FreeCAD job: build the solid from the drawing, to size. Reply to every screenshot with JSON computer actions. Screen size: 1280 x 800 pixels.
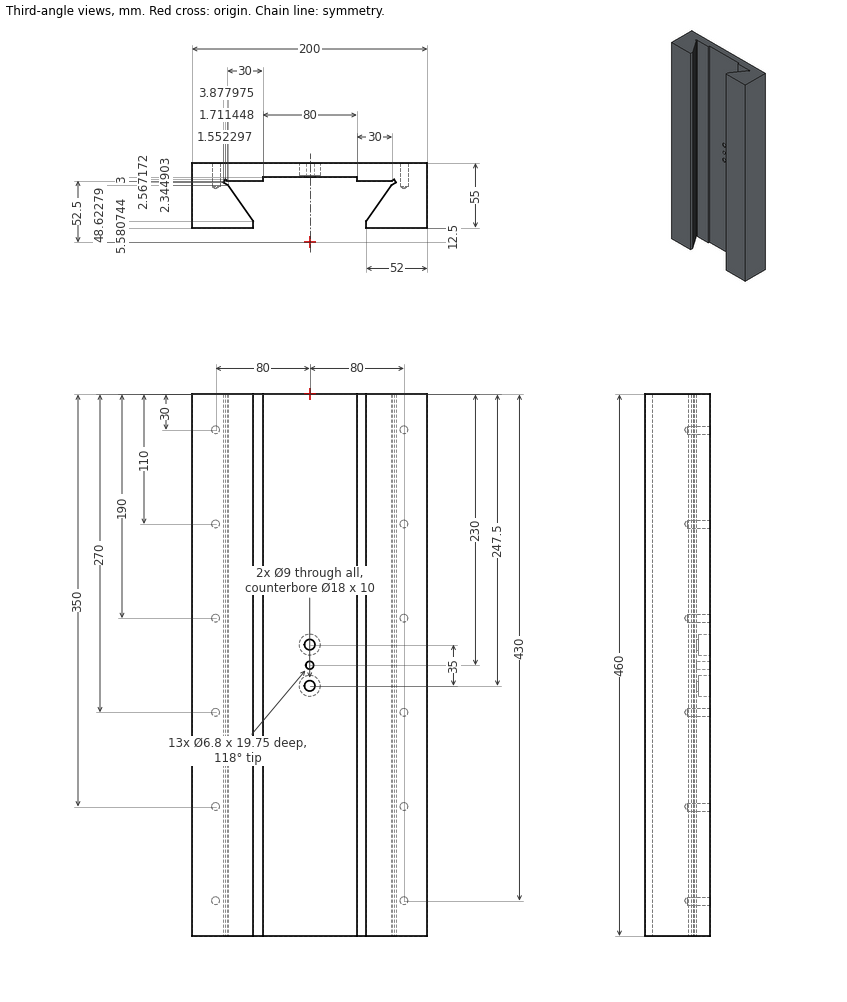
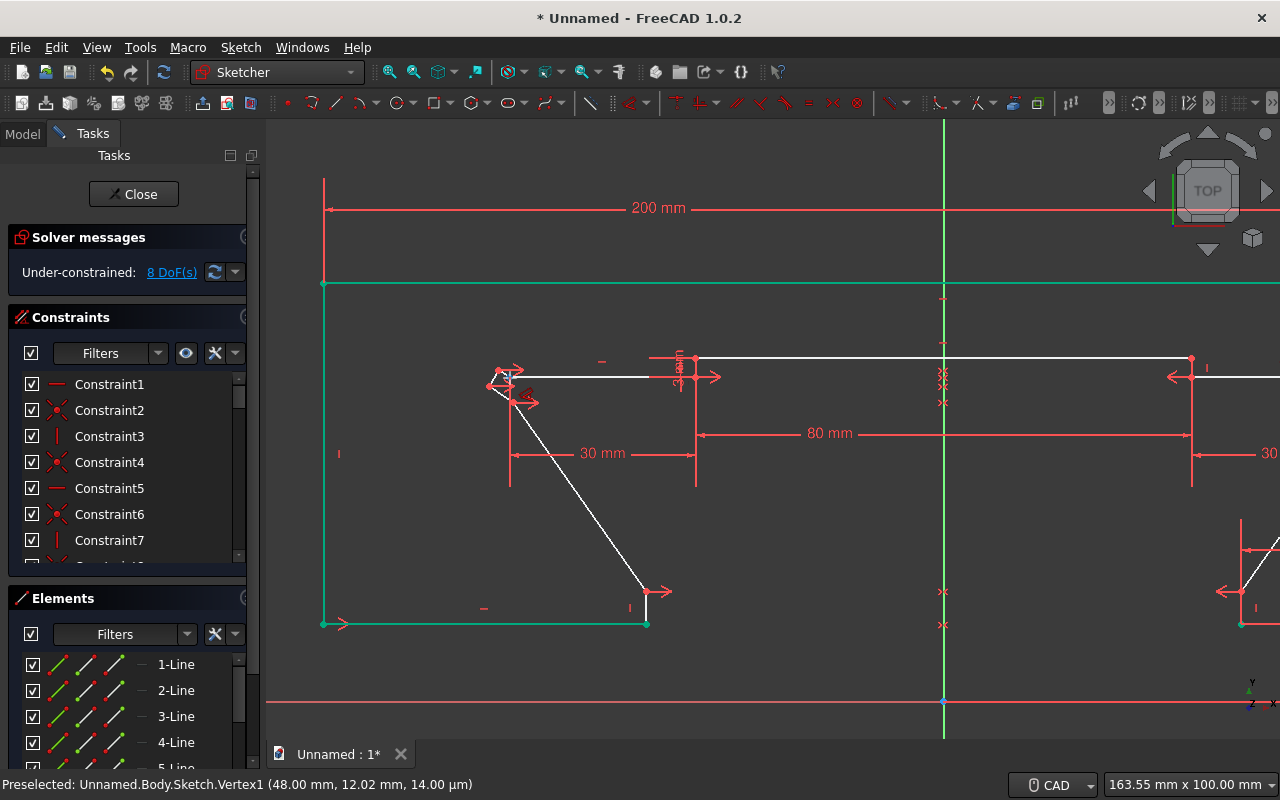
{"action": "left_click", "coordinate": [510, 377]}
{"action": "left_click", "coordinate": [476, 539]}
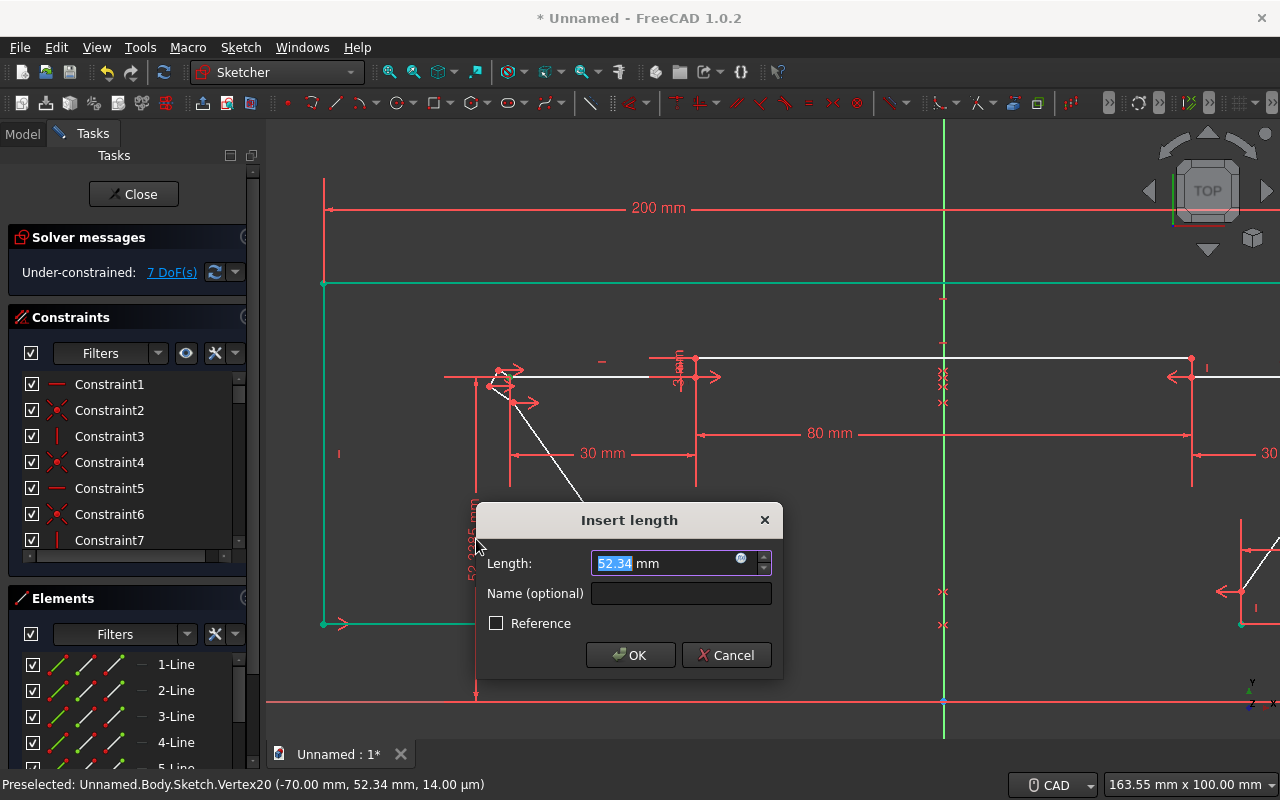
{"action": "type", "text": "52.5"}
{"action": "key", "text": "Return"}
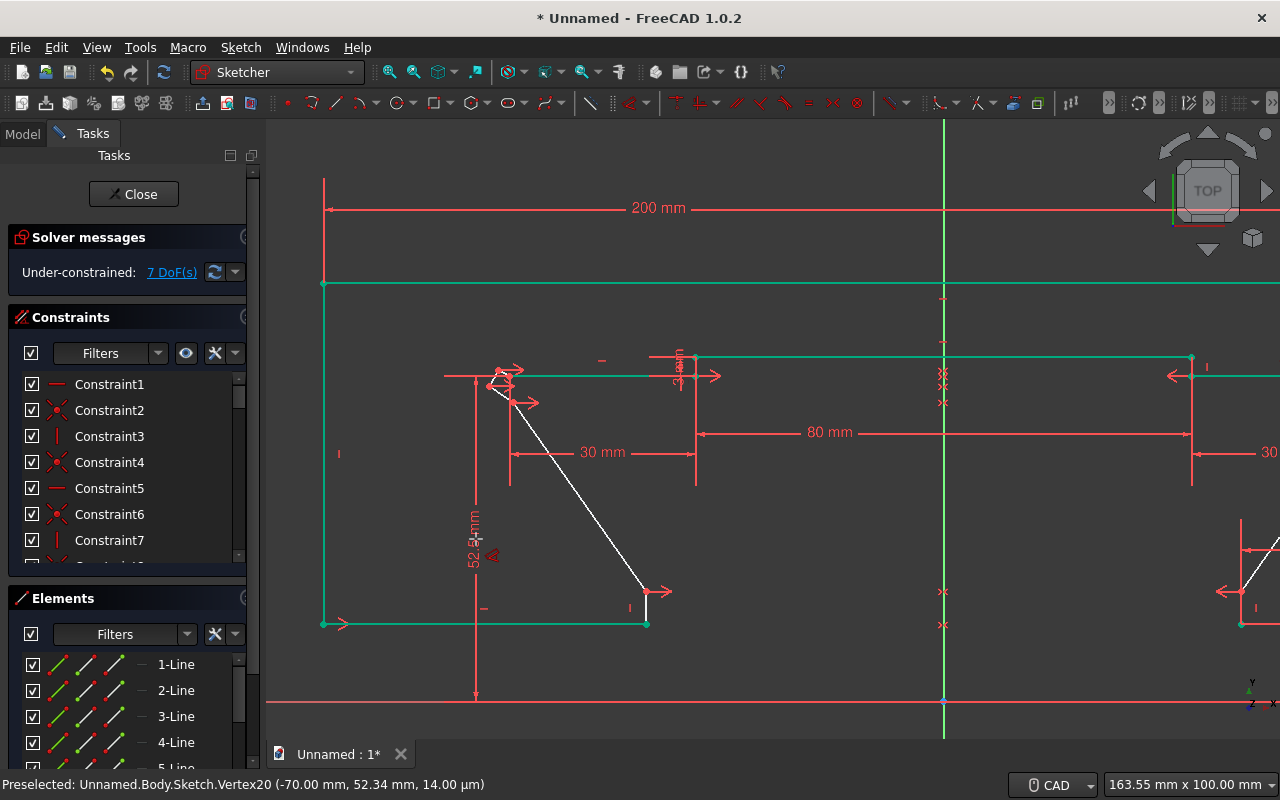
{"action": "scroll", "coordinate": [646, 614], "scroll_direction": "up", "scroll_amount": 2}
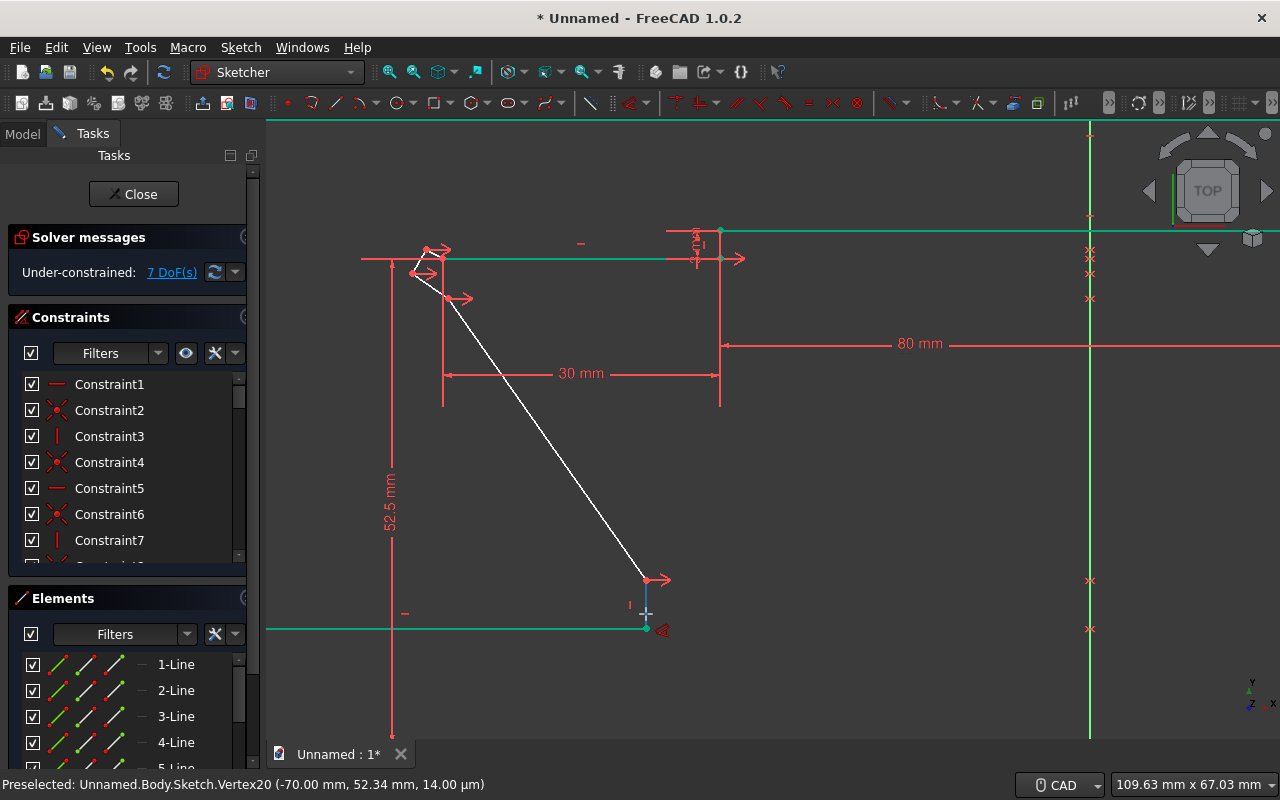
{"action": "left_click", "coordinate": [646, 614]}
{"action": "left_click", "coordinate": [612, 604]}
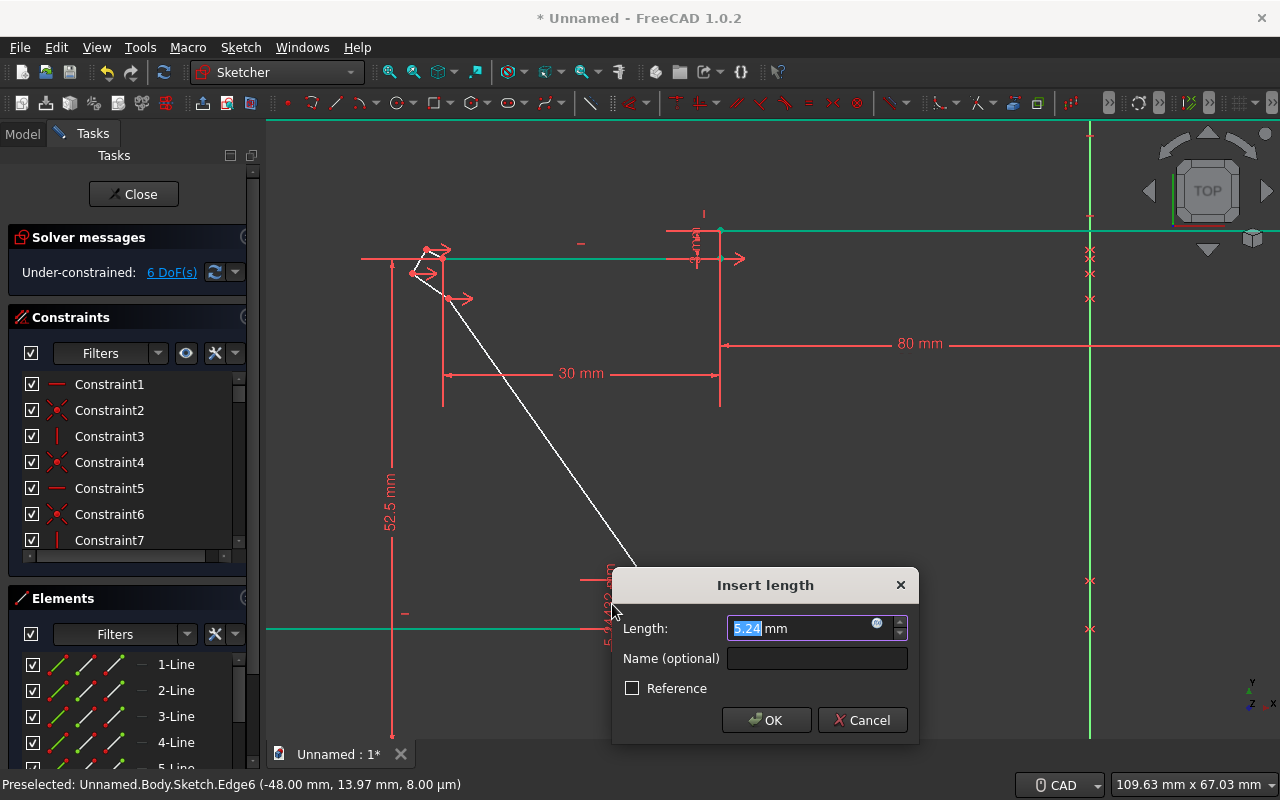
{"action": "type", "text": "5.580744"}
{"action": "key", "text": "Return"}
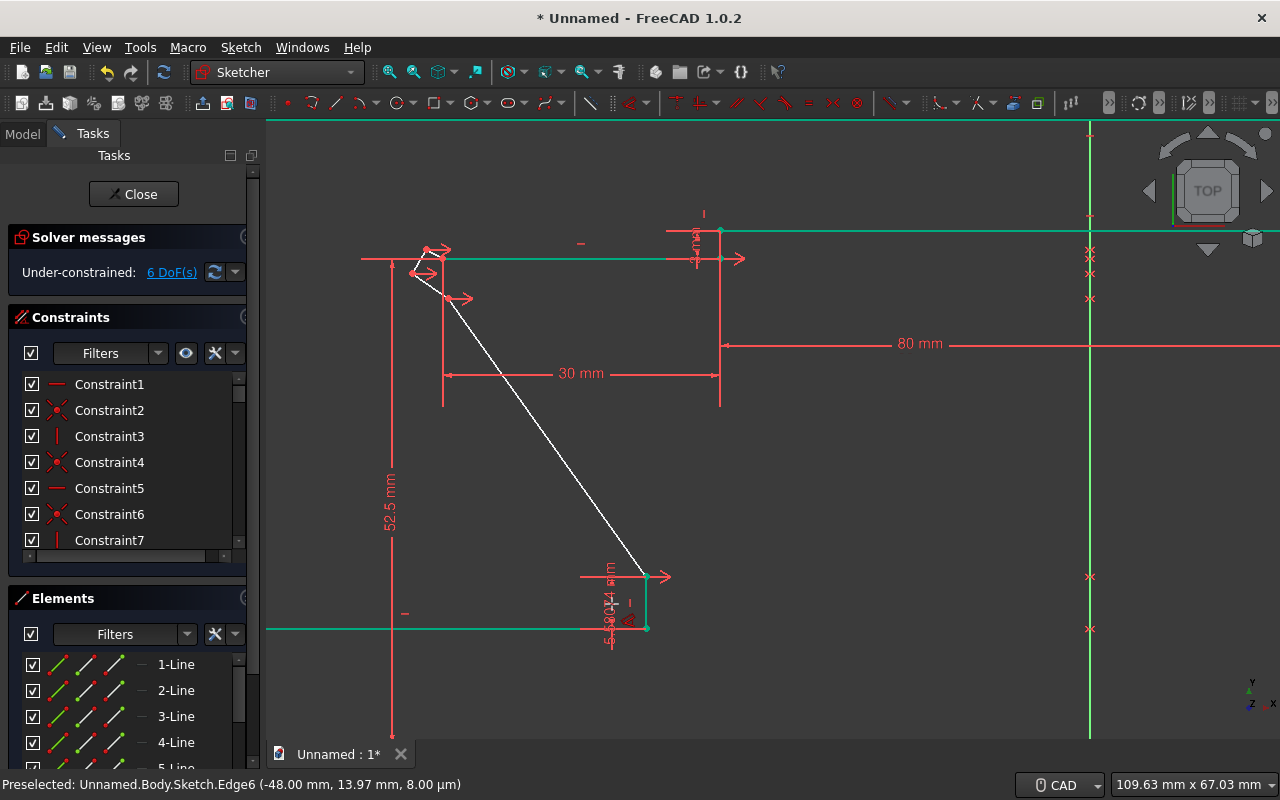
{"action": "left_click", "coordinate": [448, 299]}
{"action": "left_click", "coordinate": [414, 410]}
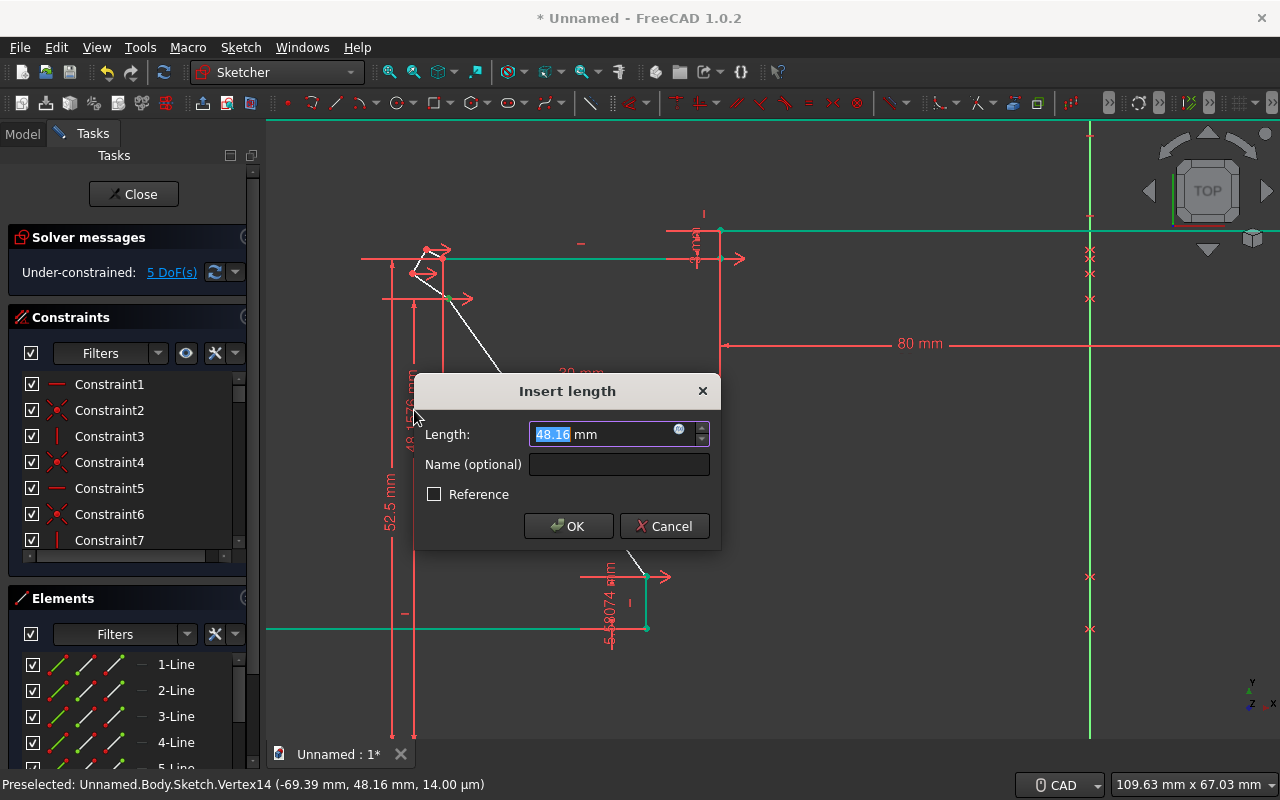
{"action": "type", "text": "48.62279"}
{"action": "key", "text": "Return"}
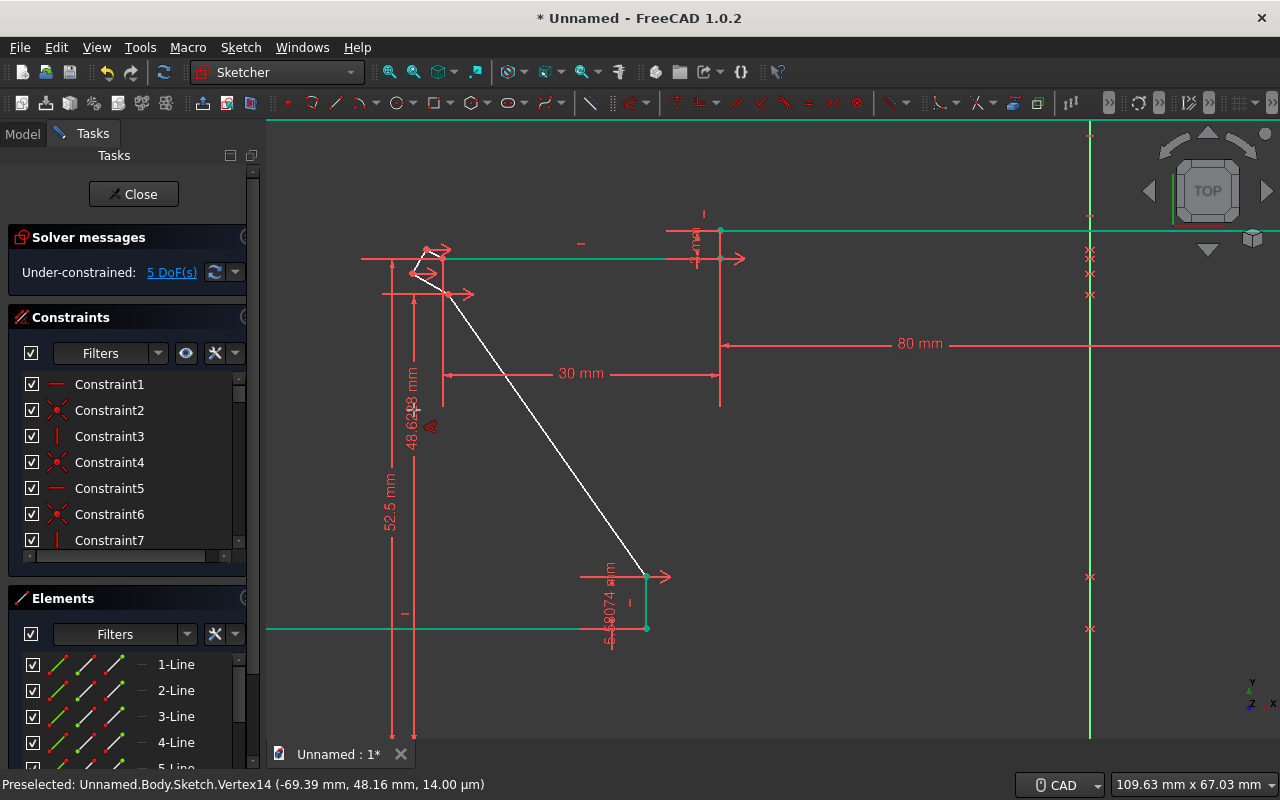
{"action": "left_click", "coordinate": [437, 288]}
{"action": "left_click", "coordinate": [438, 240]}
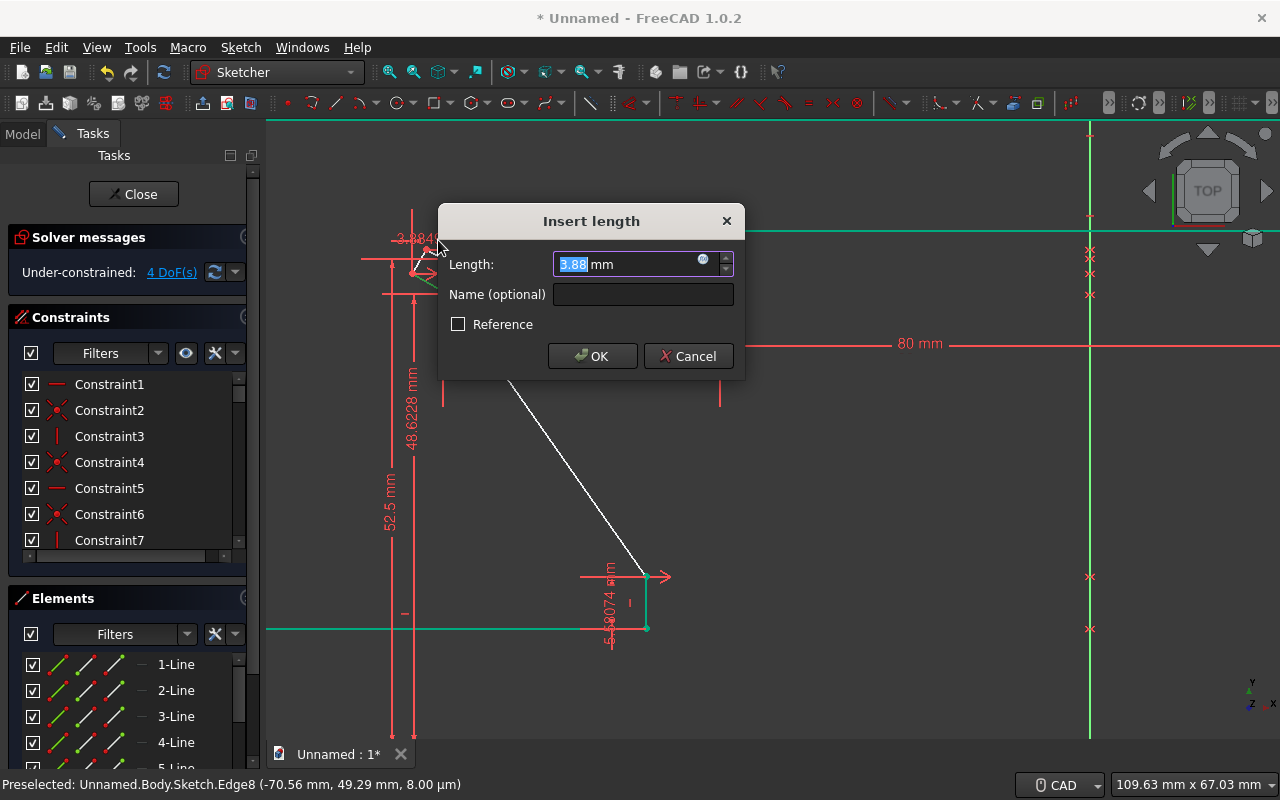
{"action": "type", "text": "3.877975"}
{"action": "key", "text": "Return"}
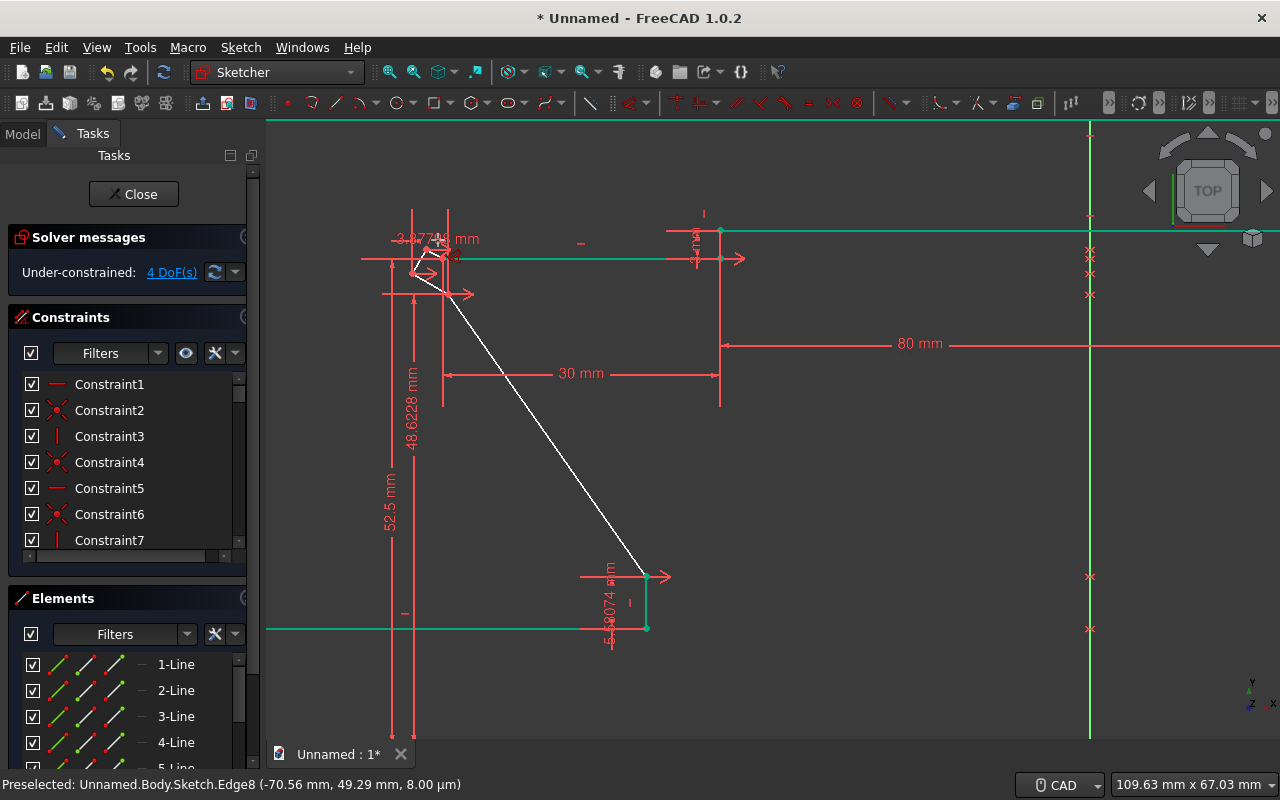
{"action": "scroll", "coordinate": [437, 288], "scroll_direction": "up", "scroll_amount": 4}